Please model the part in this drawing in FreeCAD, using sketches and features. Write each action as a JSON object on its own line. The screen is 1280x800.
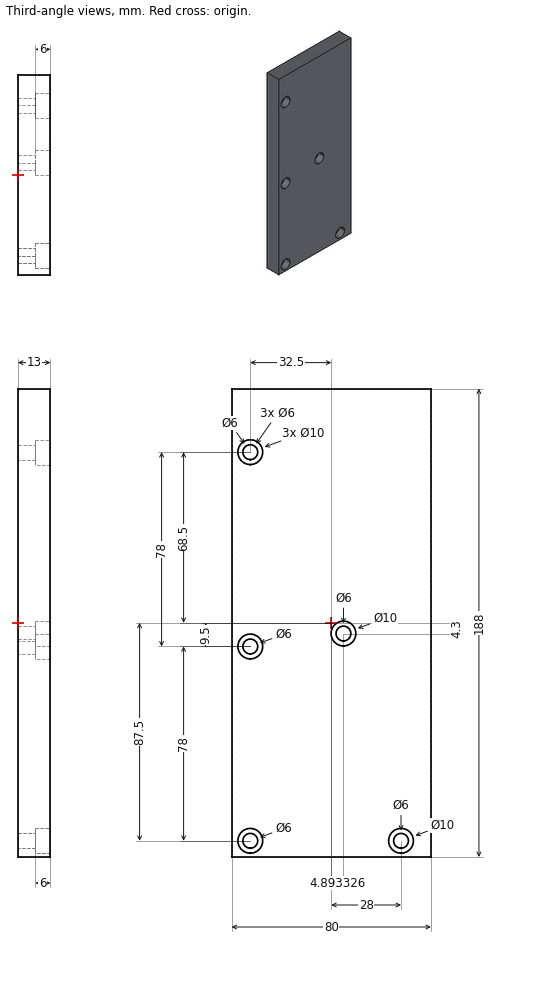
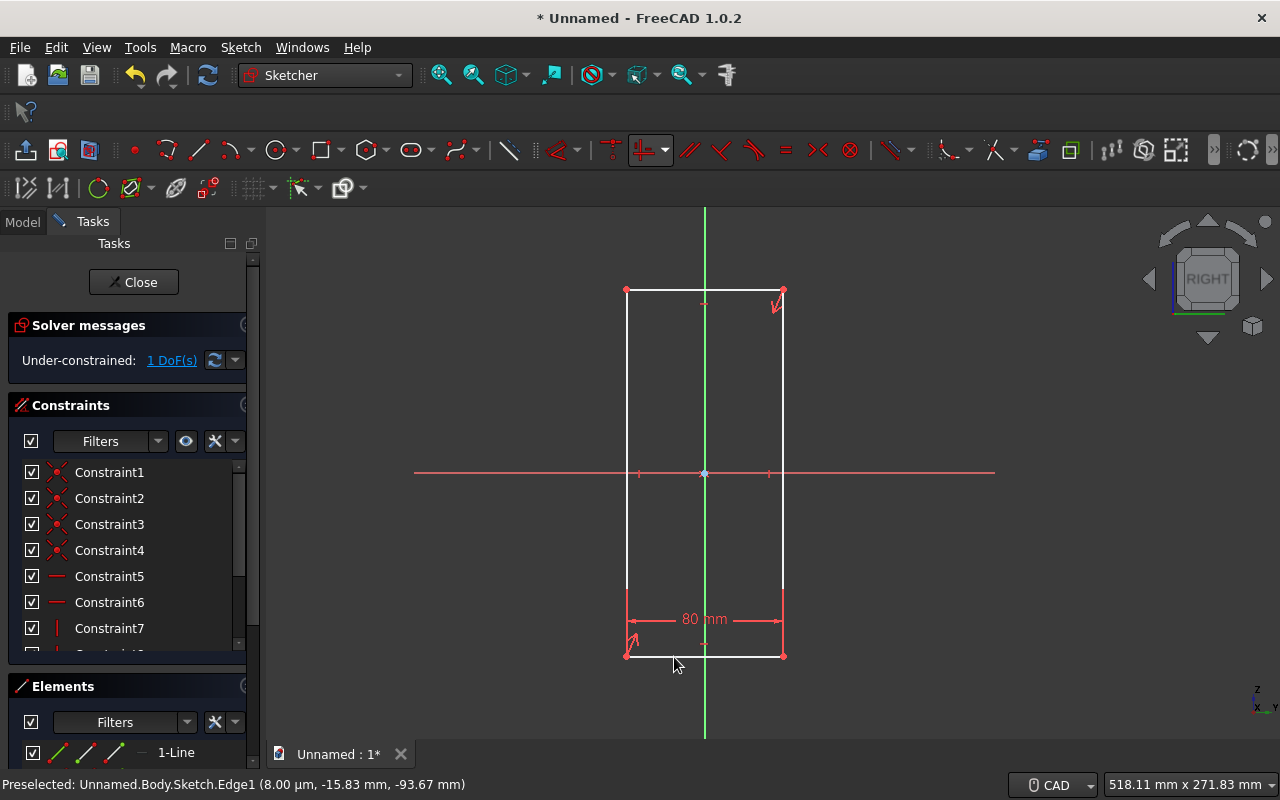
{"action": "left_click", "coordinate": [783, 547]}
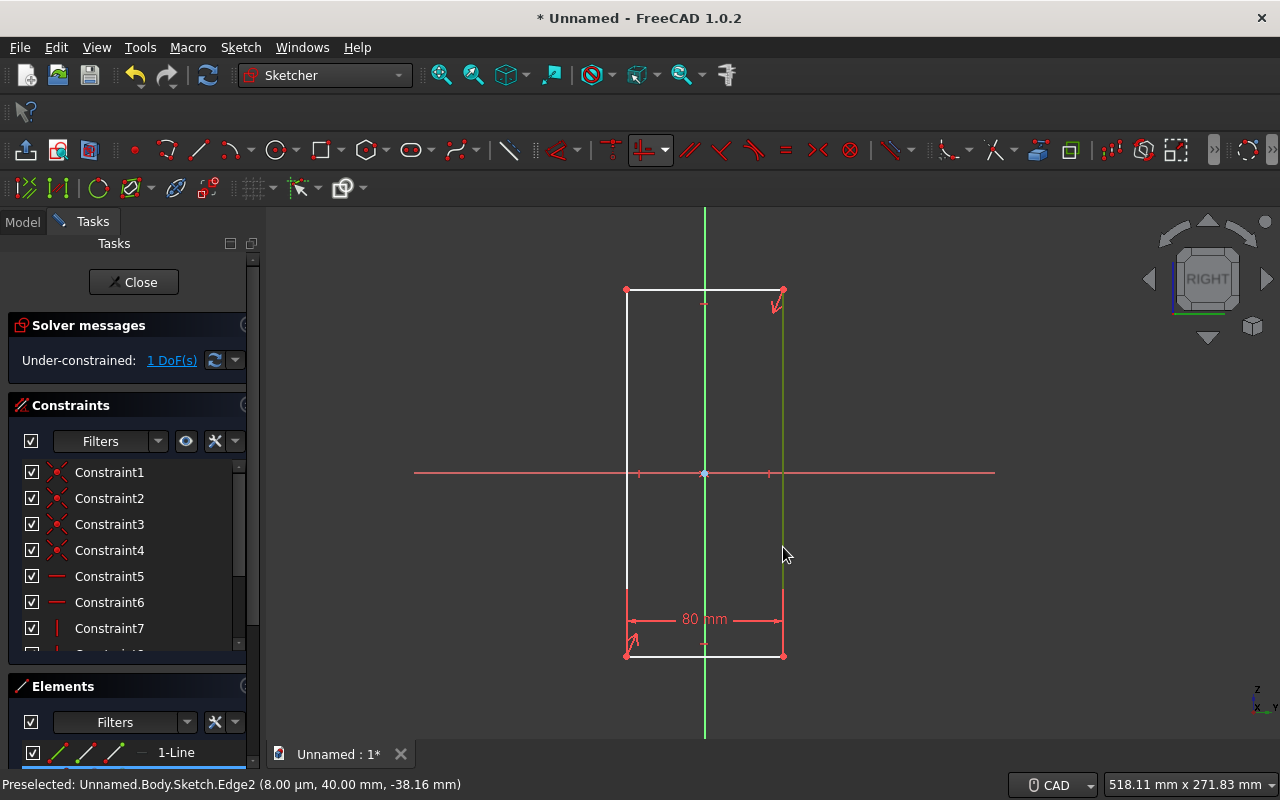
{"action": "key", "text": "i"}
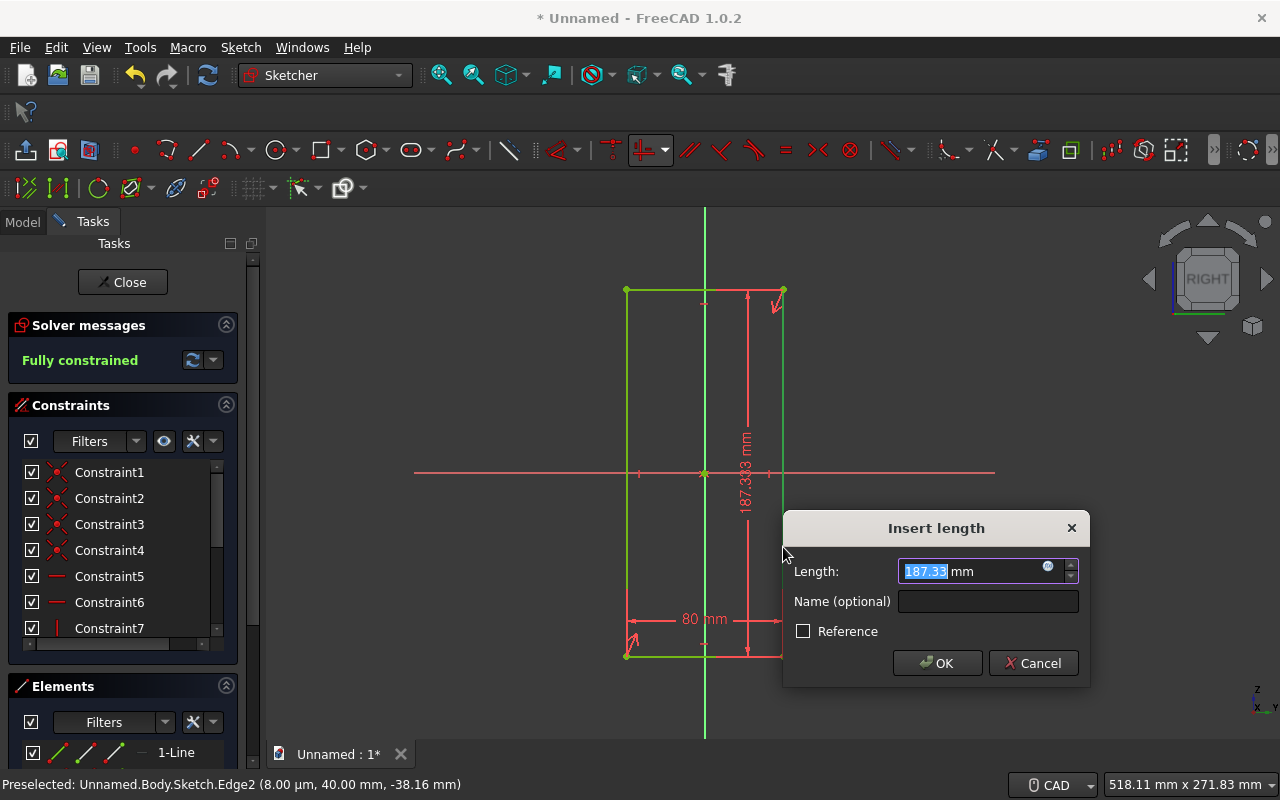
{"action": "type", "text": "188"}
{"action": "key", "text": "Return"}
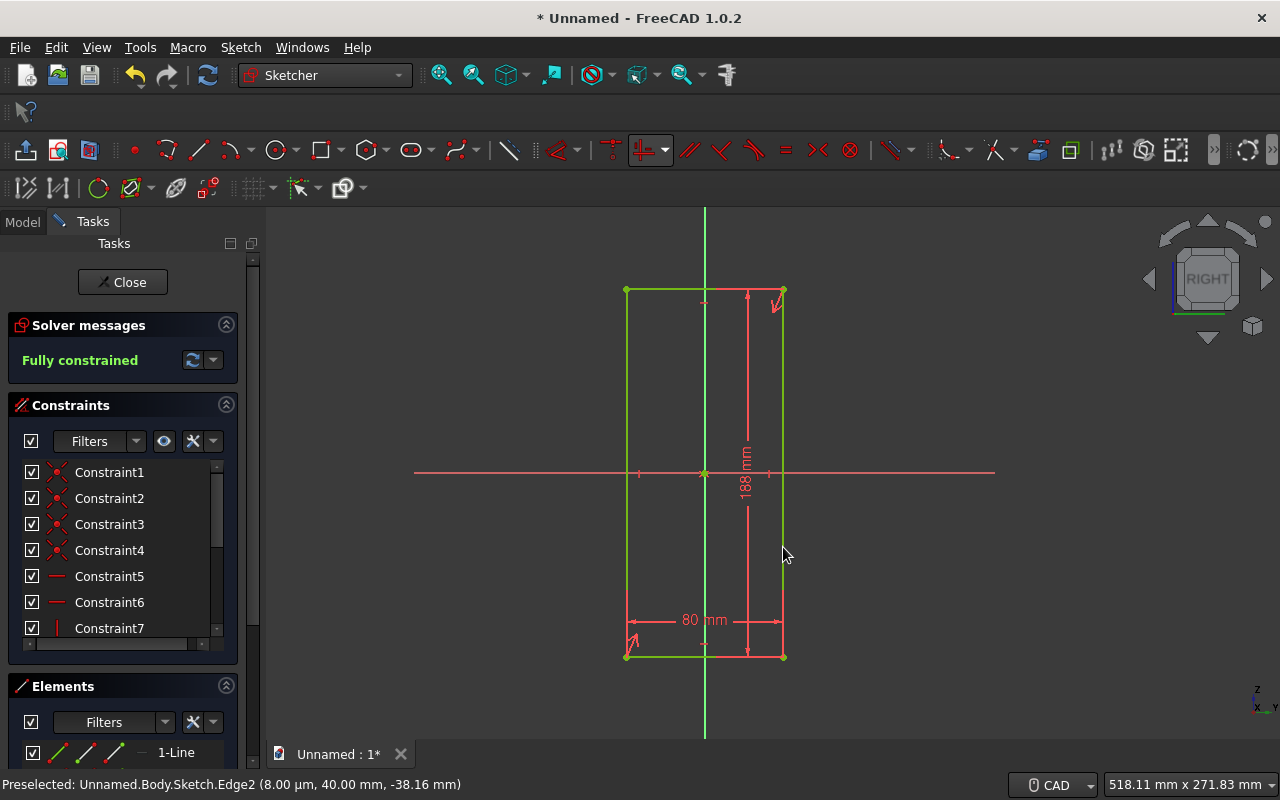
{"action": "left_click", "coordinate": [123, 282]}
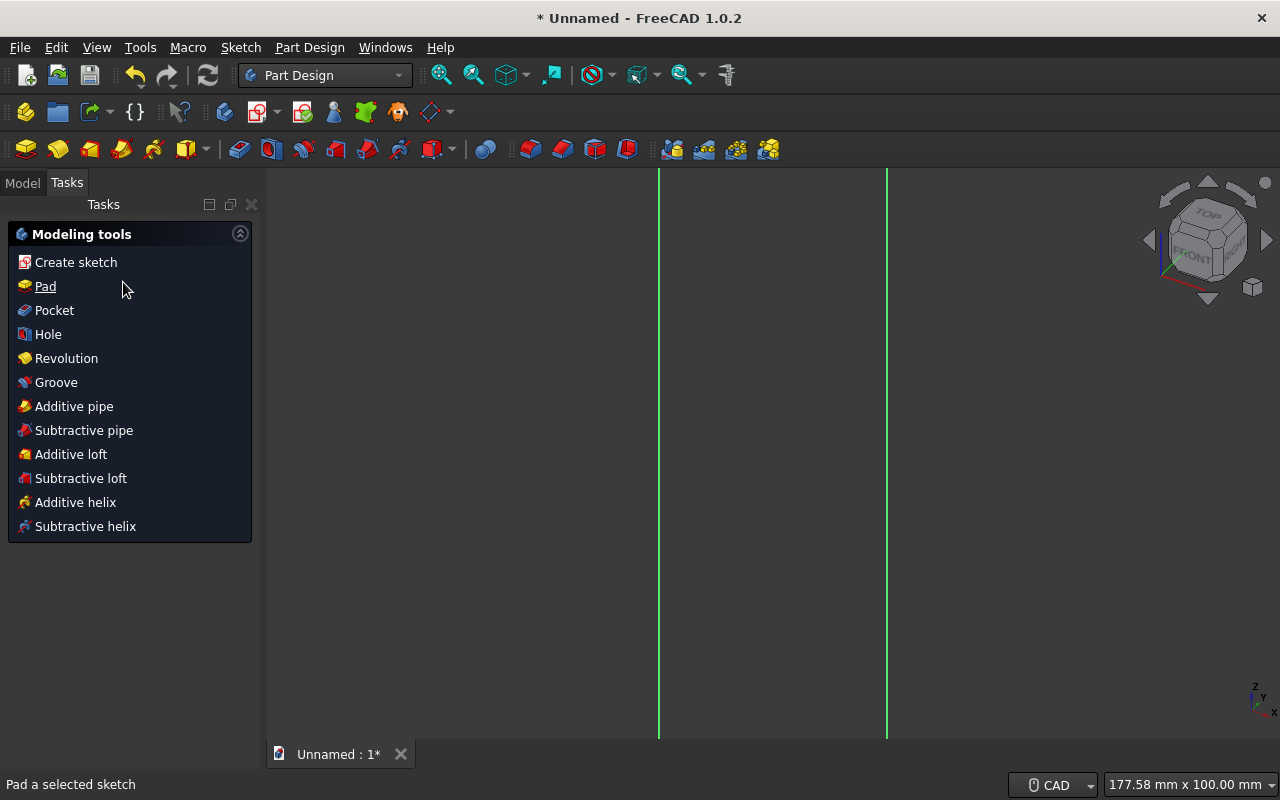
{"action": "left_click", "coordinate": [26, 150]}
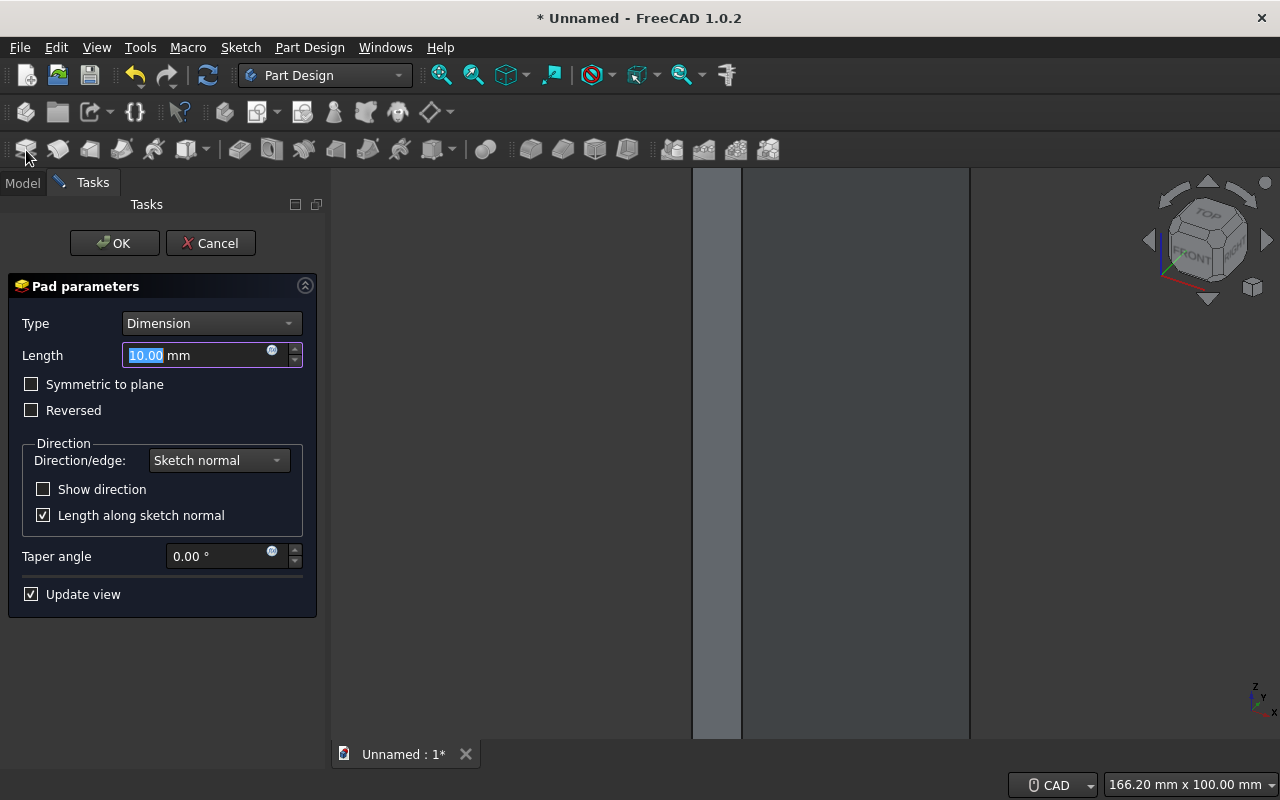
{"action": "type", "text": "13"}
{"action": "key", "text": "Tab"}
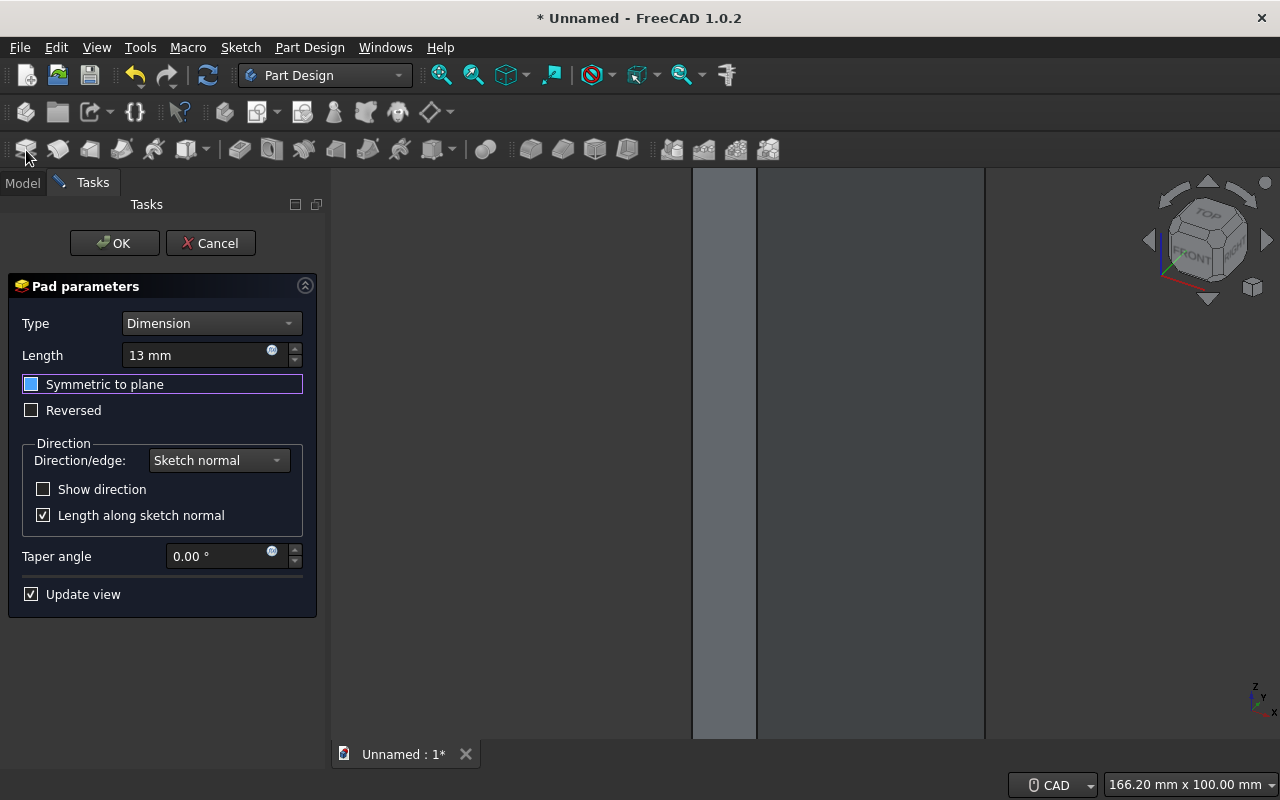
{"action": "left_click", "coordinate": [115, 243]}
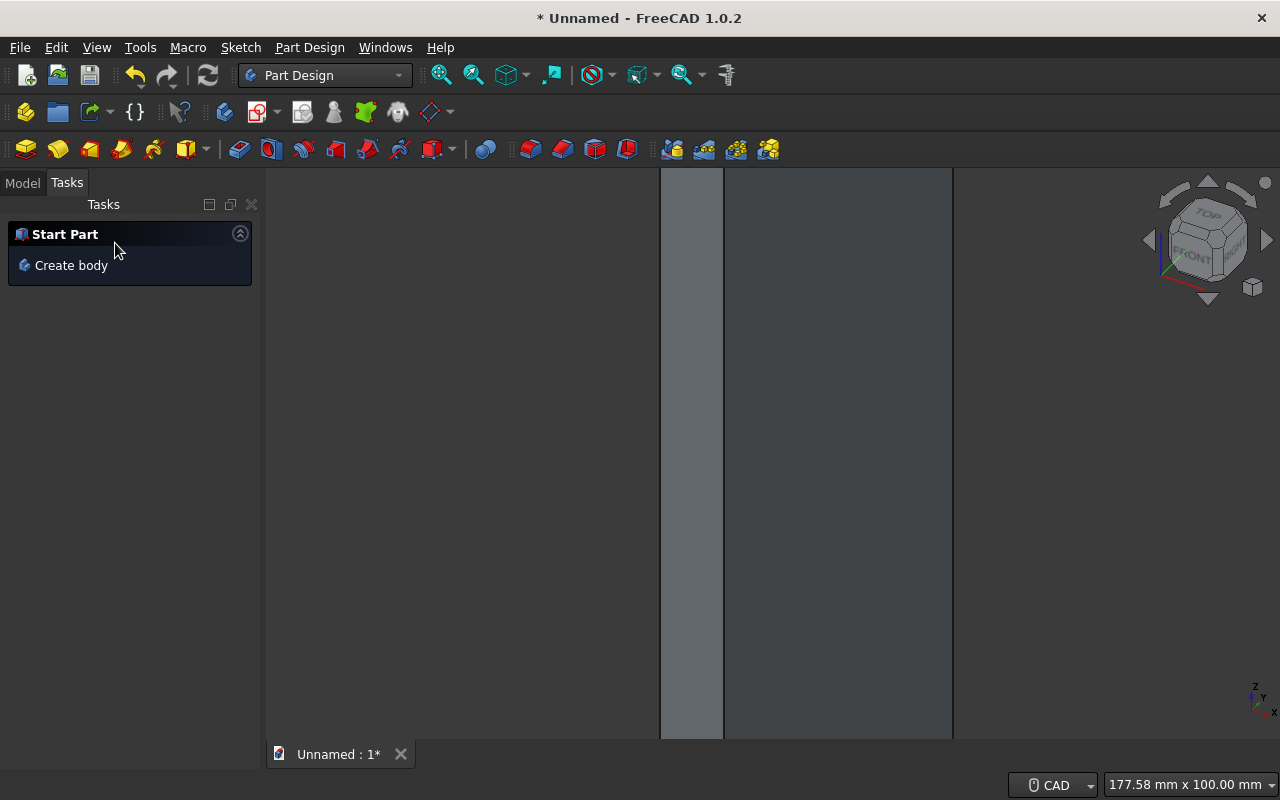
{"action": "left_click", "coordinate": [442, 76]}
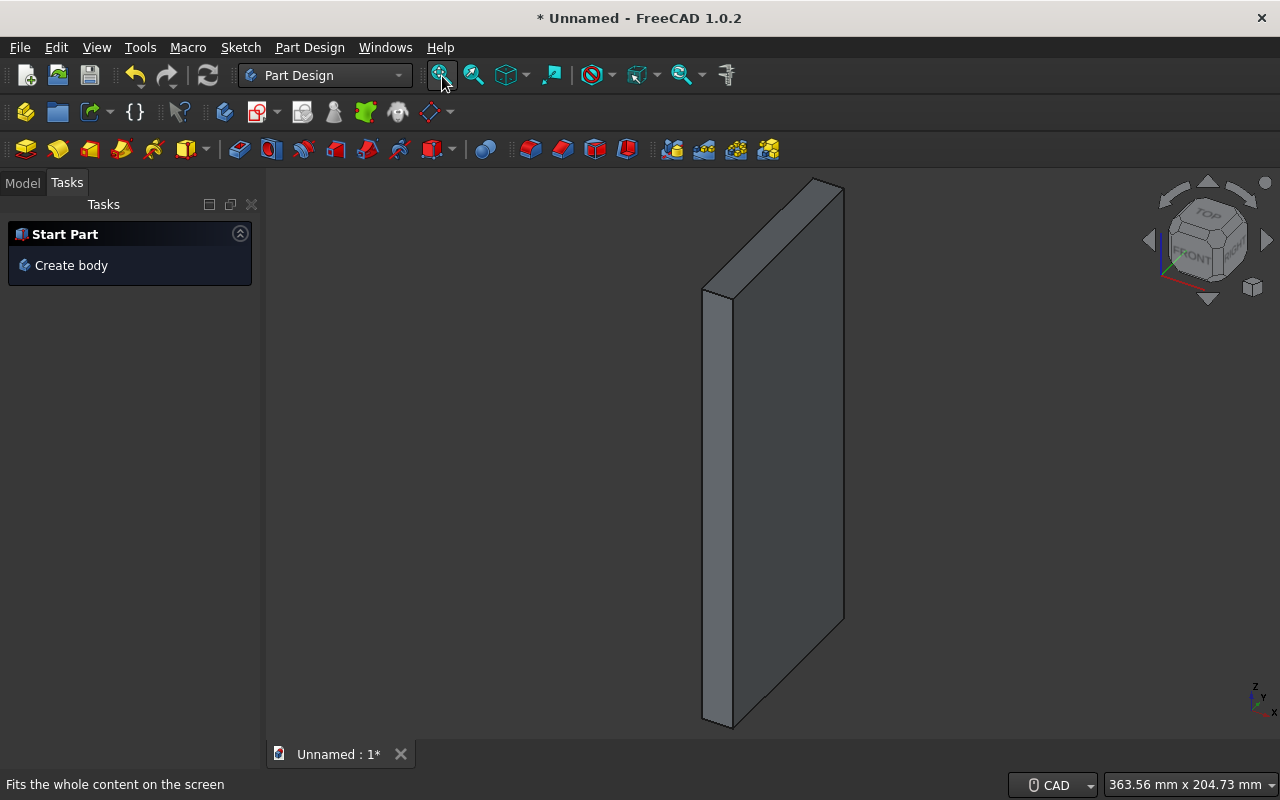
{"action": "left_click", "coordinate": [789, 580]}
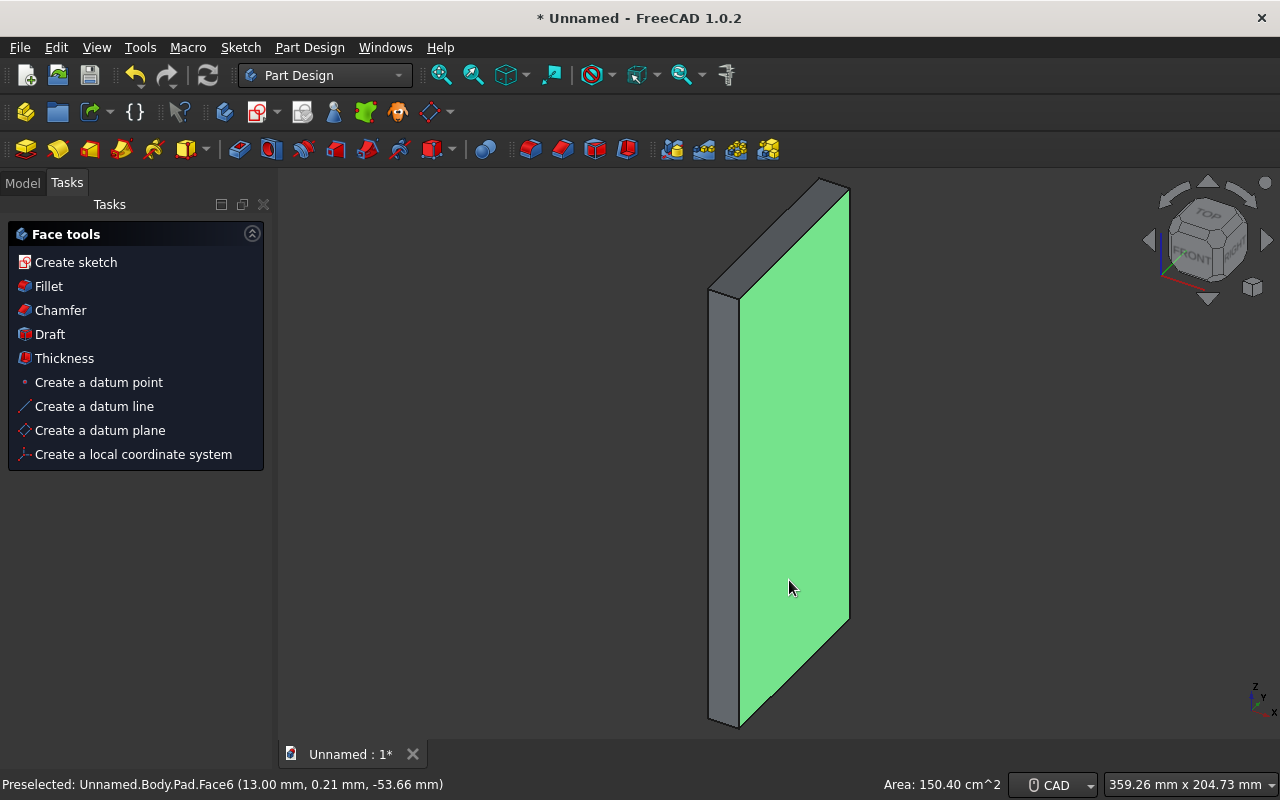
{"action": "left_click", "coordinate": [258, 112]}